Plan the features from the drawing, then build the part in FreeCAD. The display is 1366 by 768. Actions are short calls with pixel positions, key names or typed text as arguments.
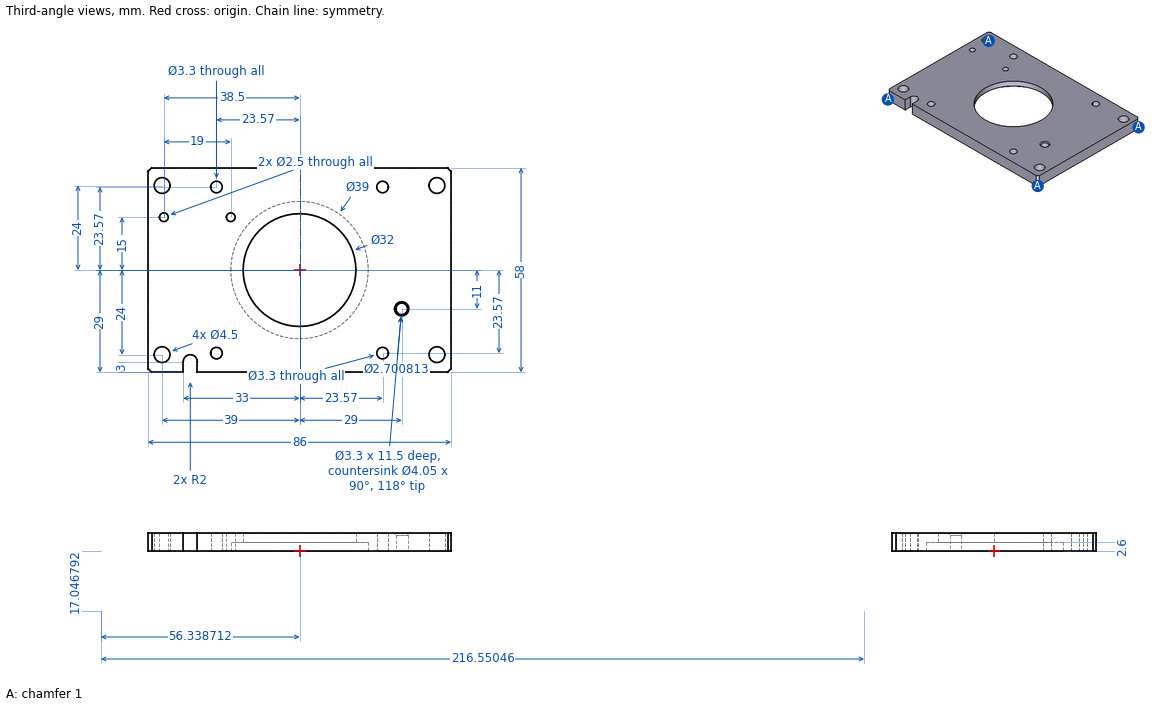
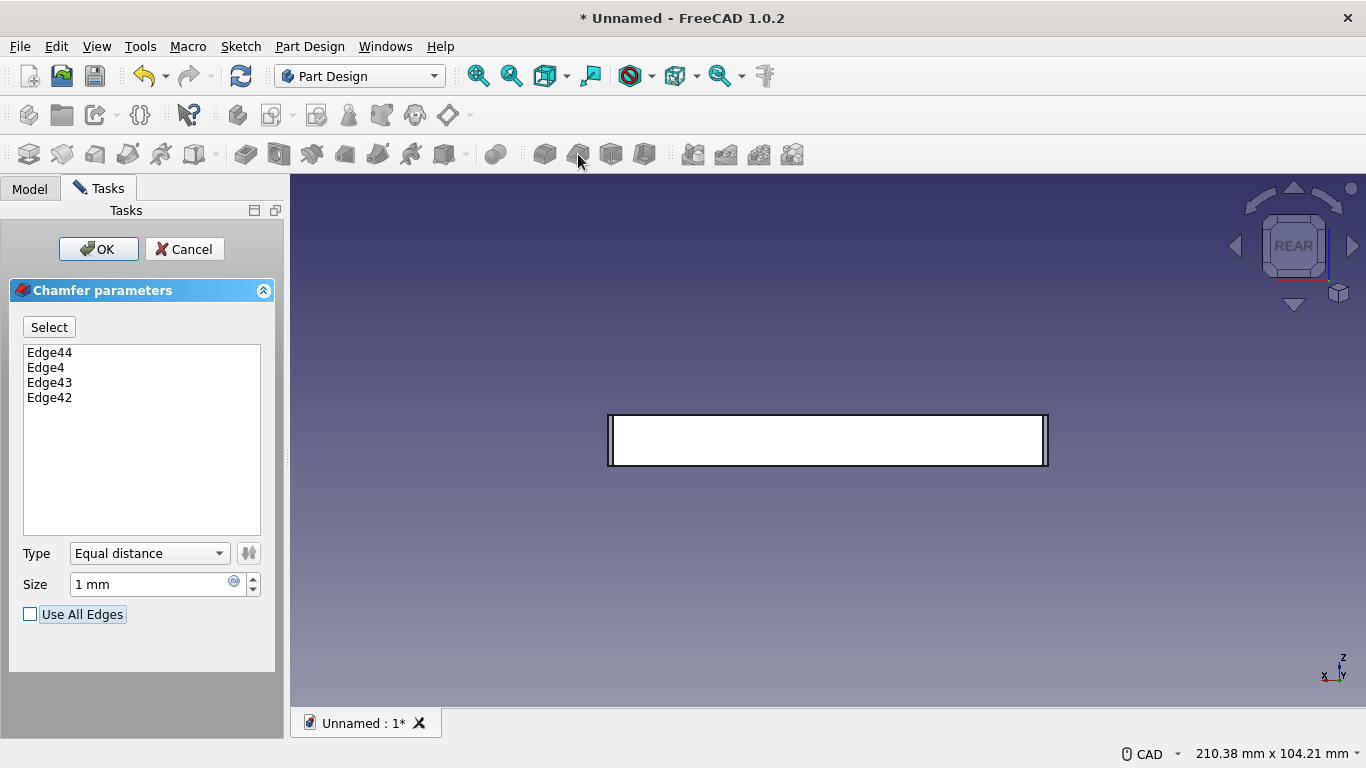
click(99, 249)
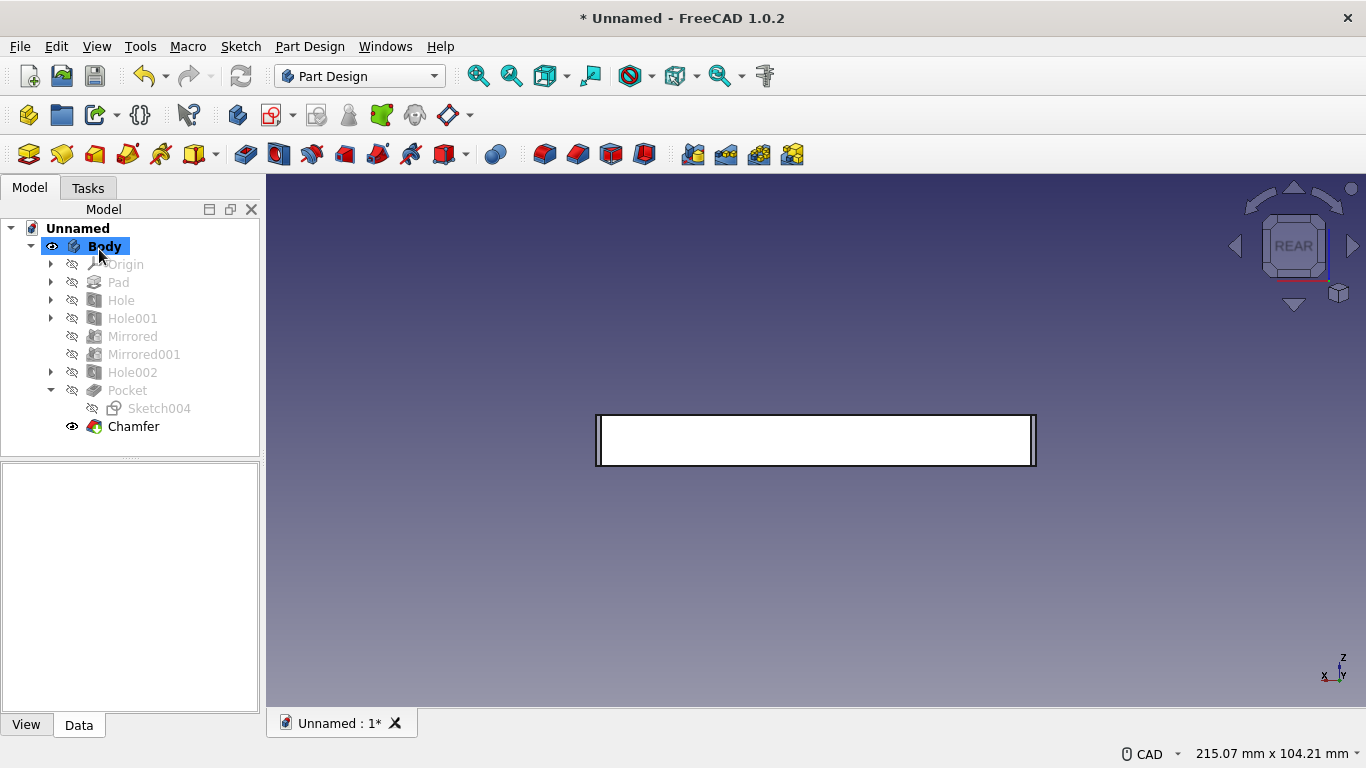
click(479, 76)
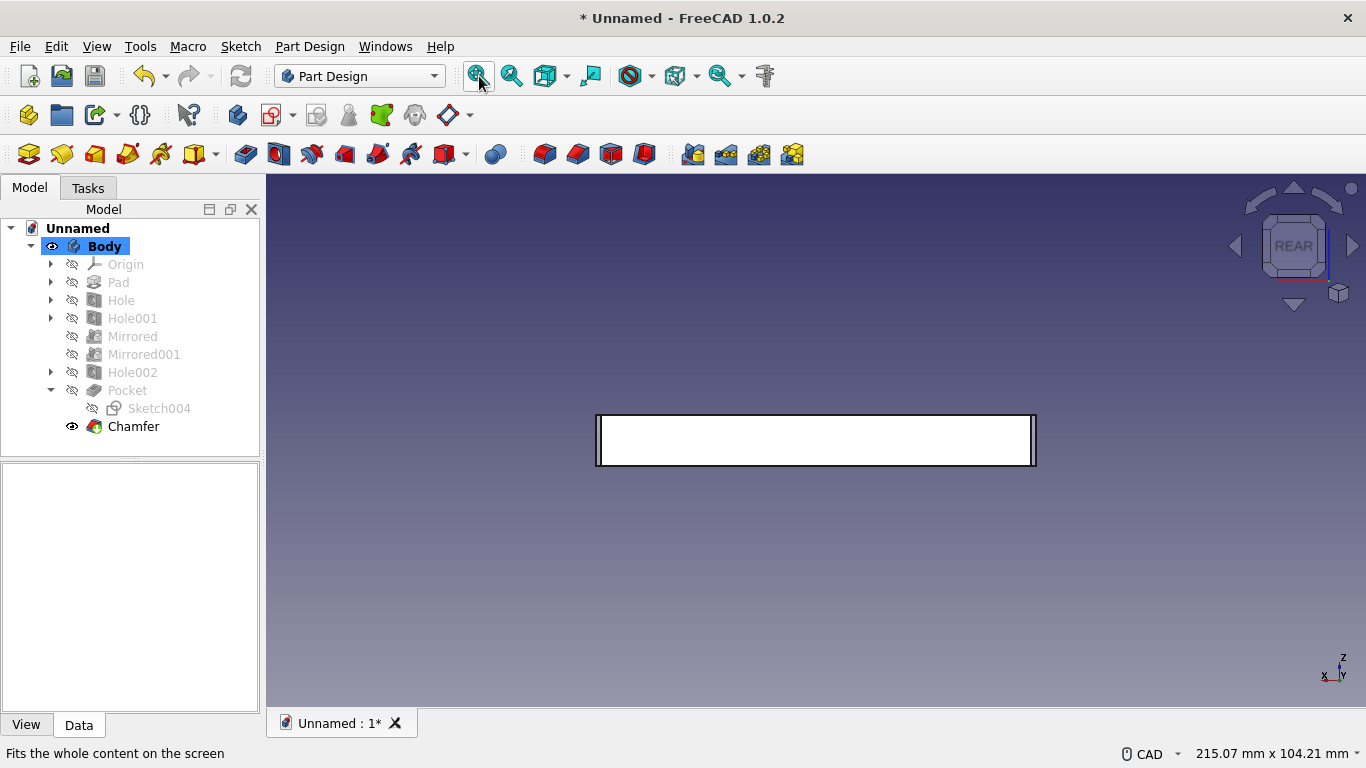
click(632, 440)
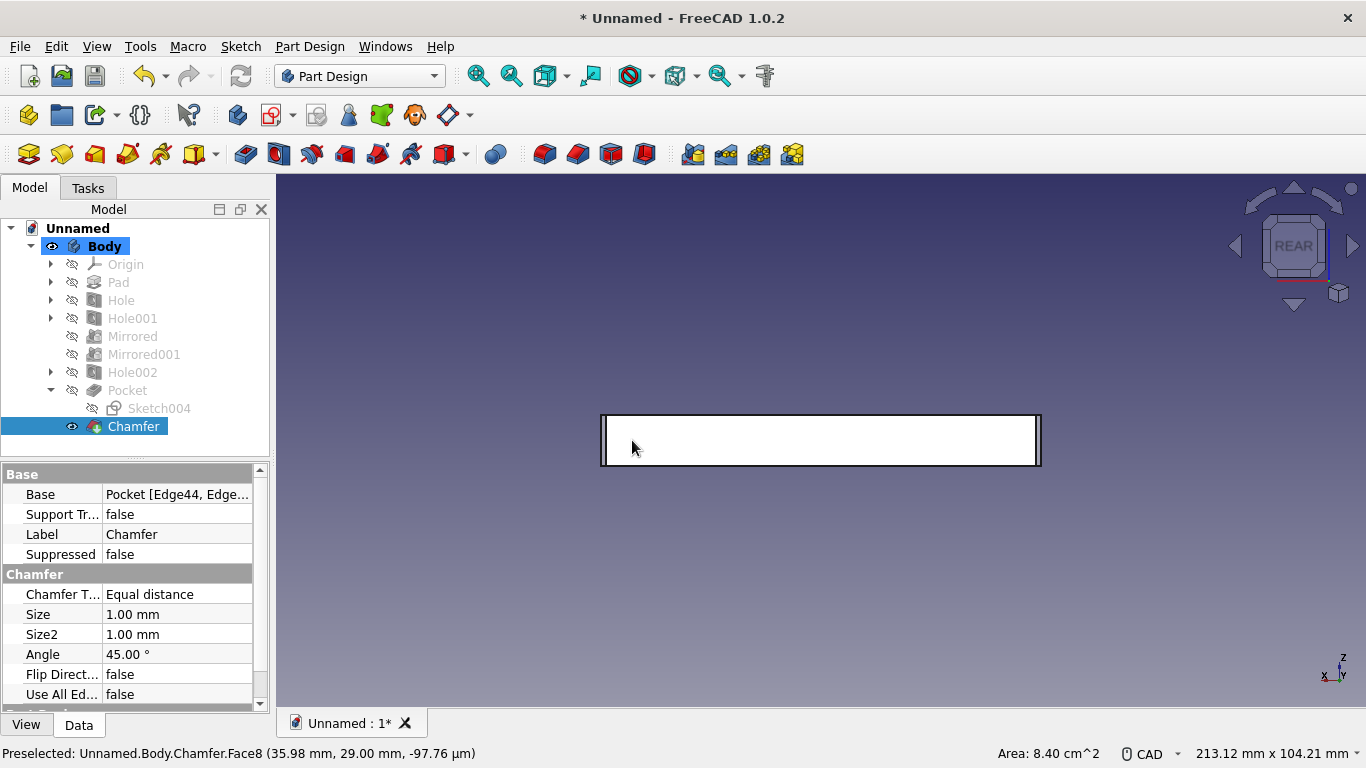
click(270, 116)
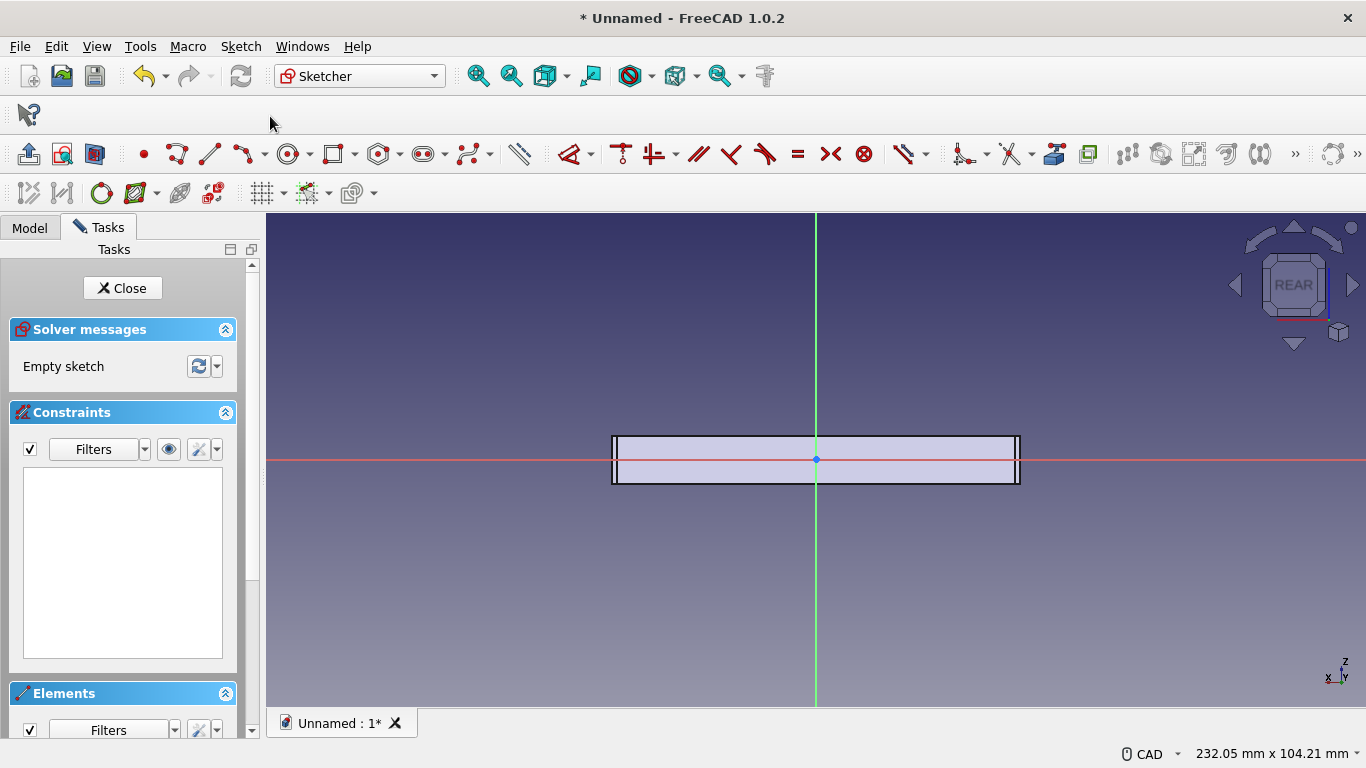
scroll(1109, 378, down, 2)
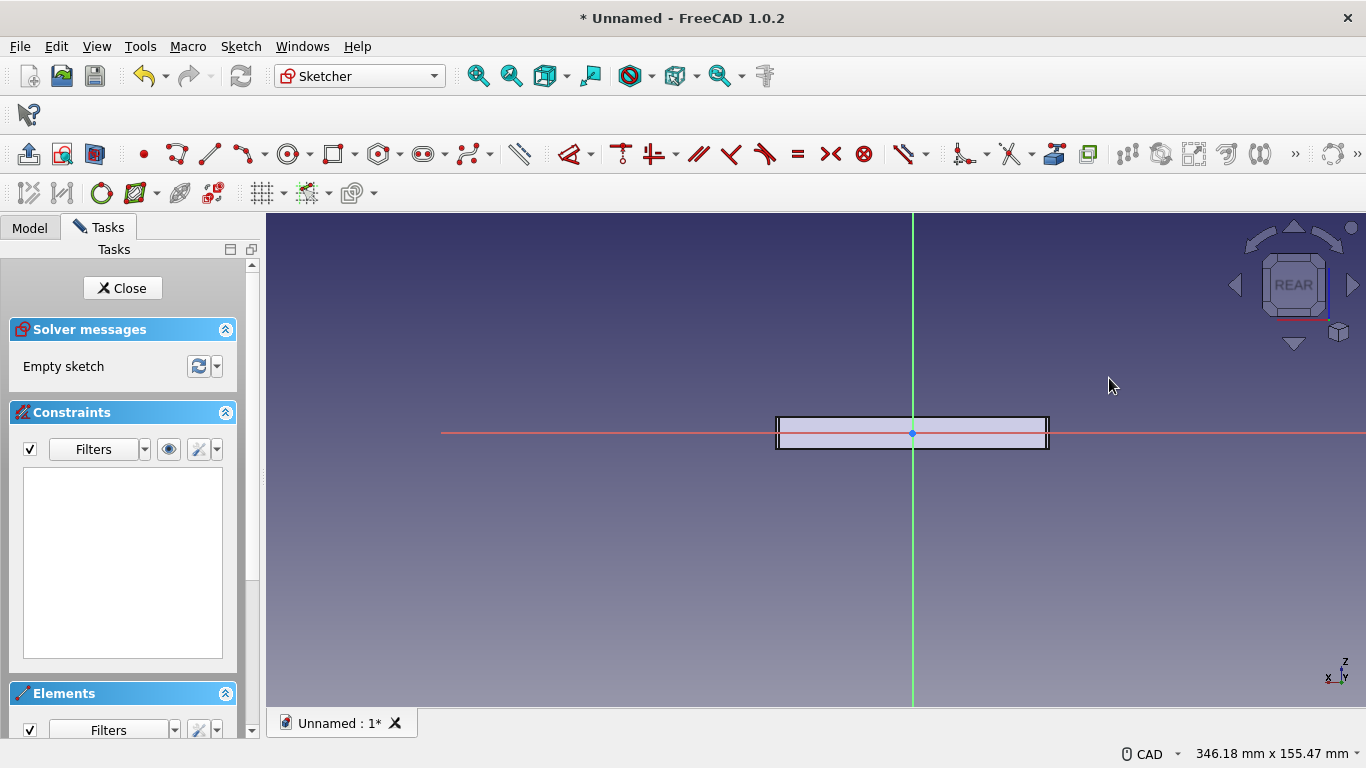
key(g)
key(r)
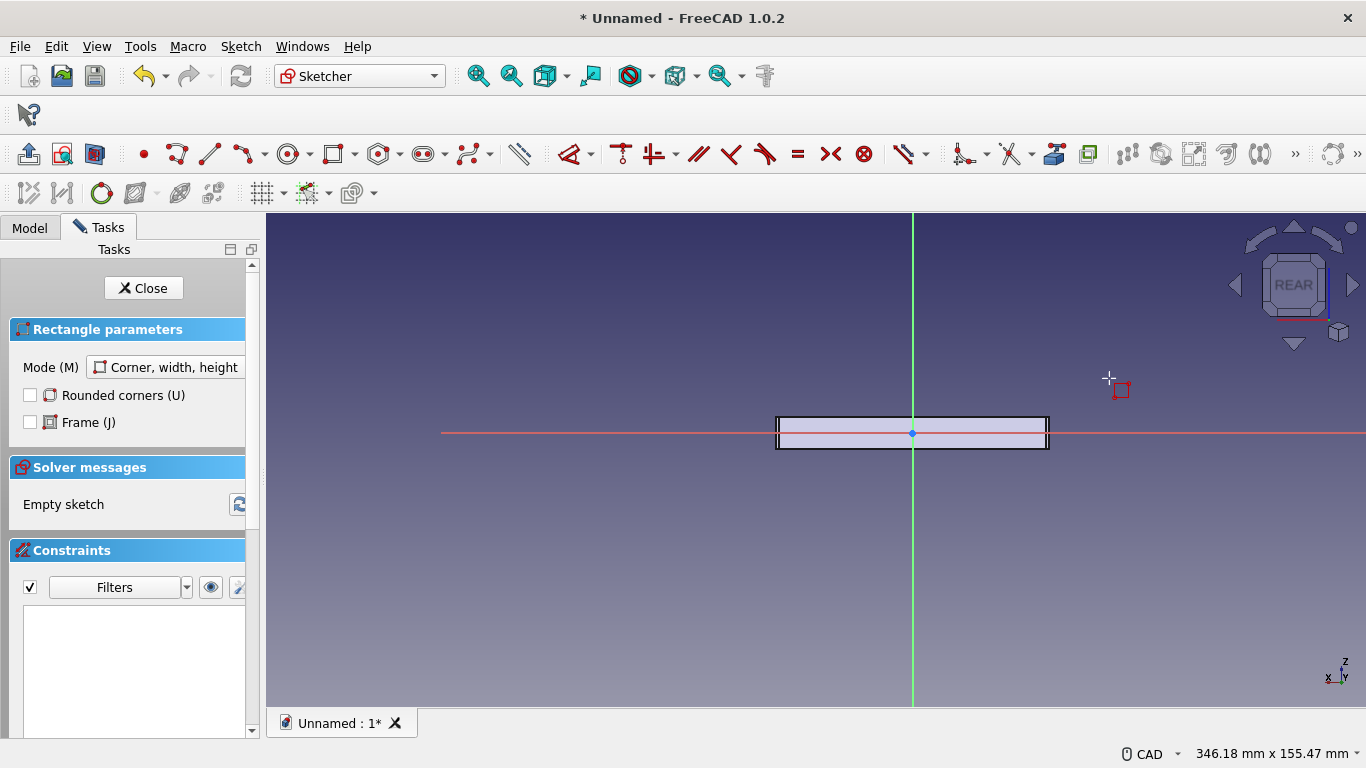
click(404, 433)
move(1092, 487)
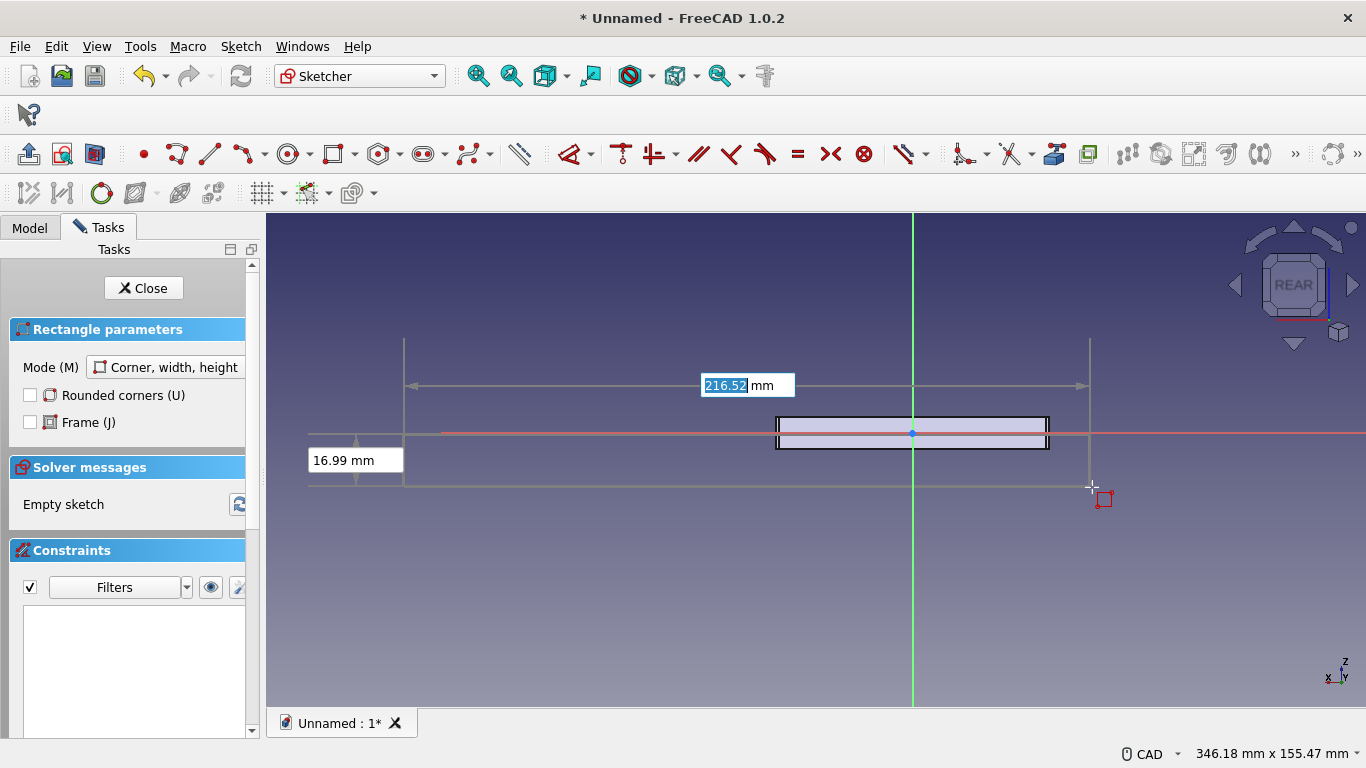
text(216.55046)
key(Tab)
text(17.046792)
key(Return)
key(Escape)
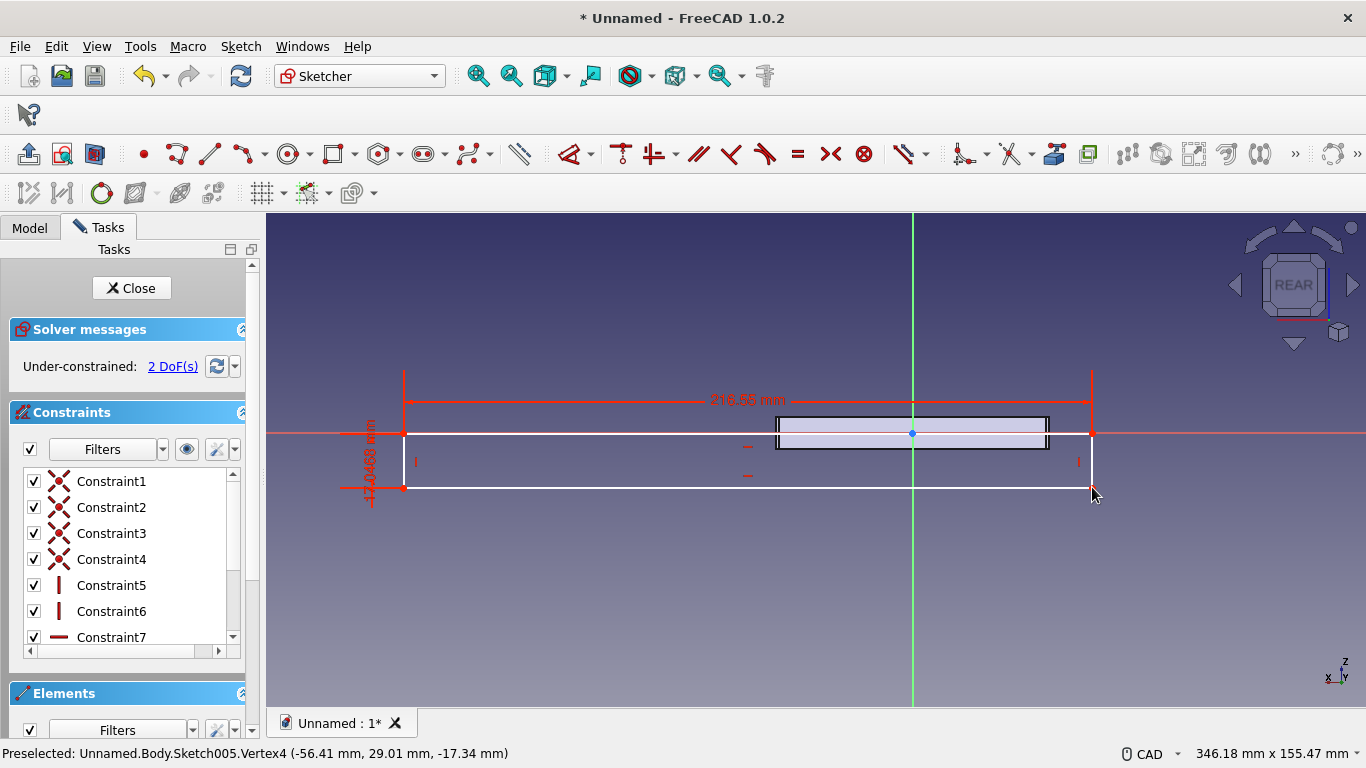
click(404, 434)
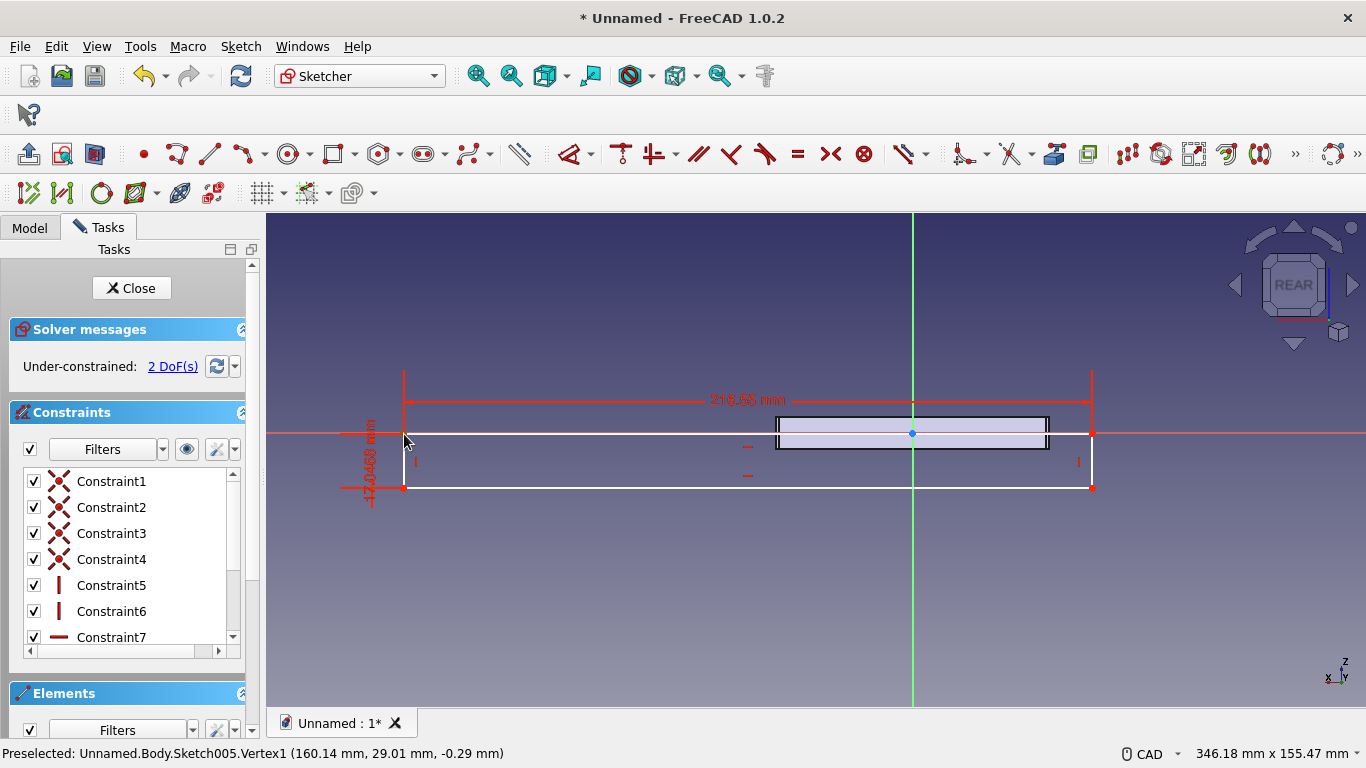
click(359, 433)